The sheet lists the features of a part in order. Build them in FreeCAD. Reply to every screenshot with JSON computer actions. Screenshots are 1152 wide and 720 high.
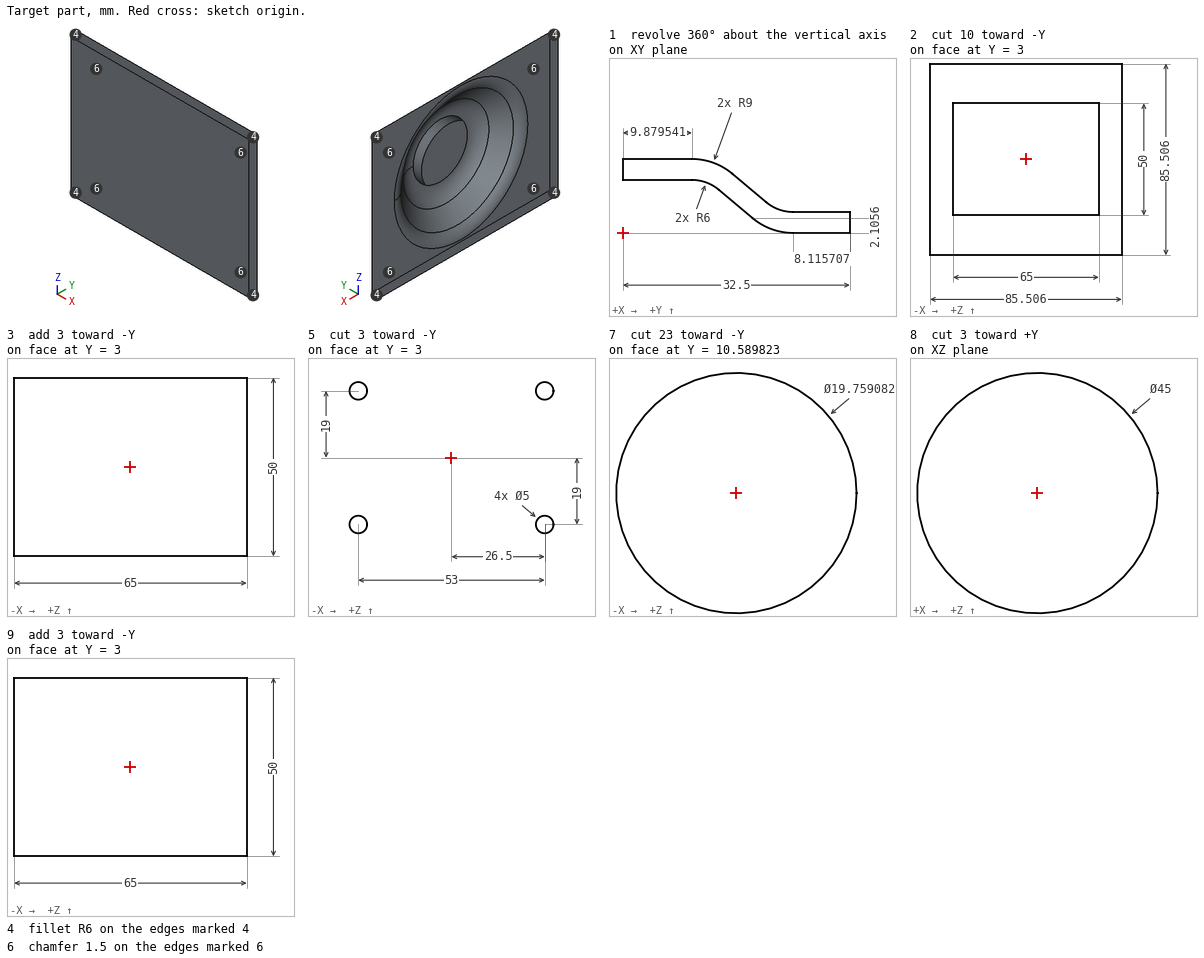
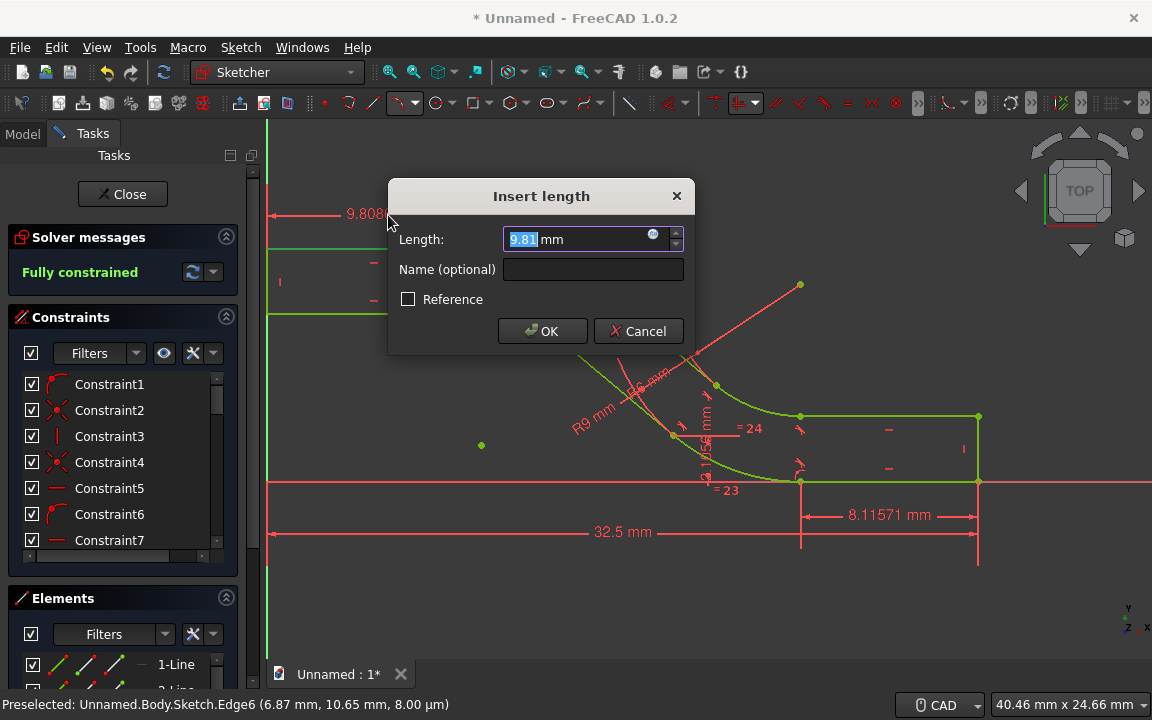
{"action": "type", "text": "9.879541"}
{"action": "key", "text": "Return"}
{"action": "key", "text": "Escape"}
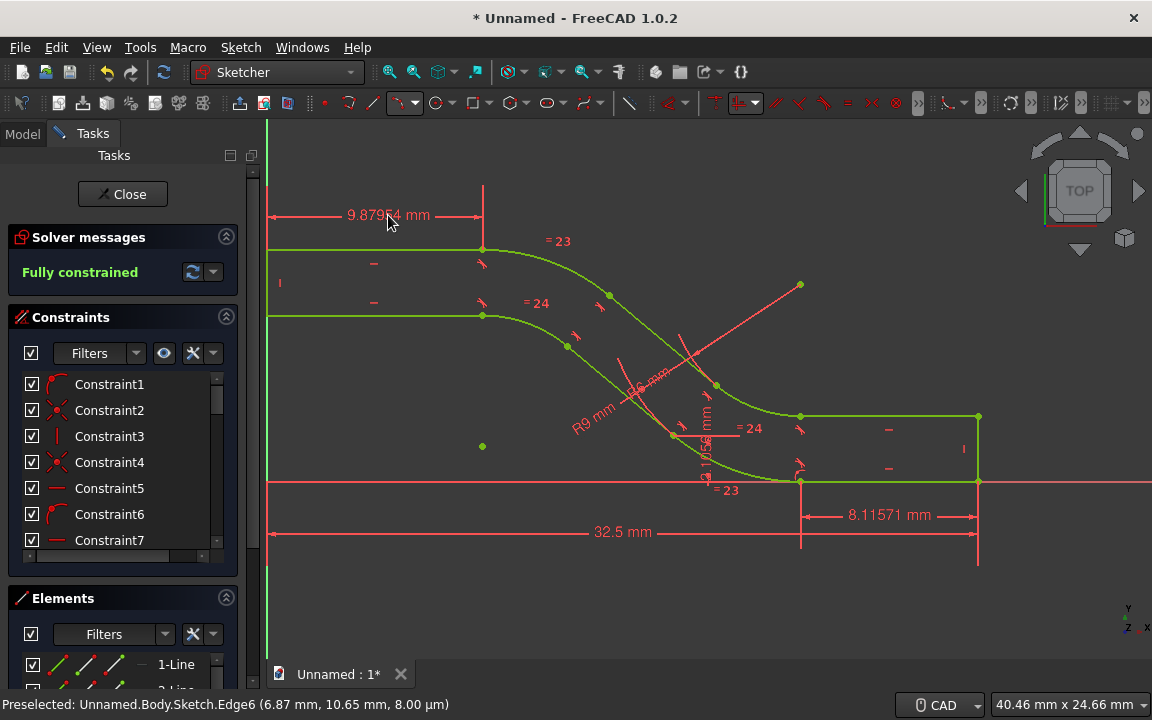
{"action": "left_click", "coordinate": [123, 194]}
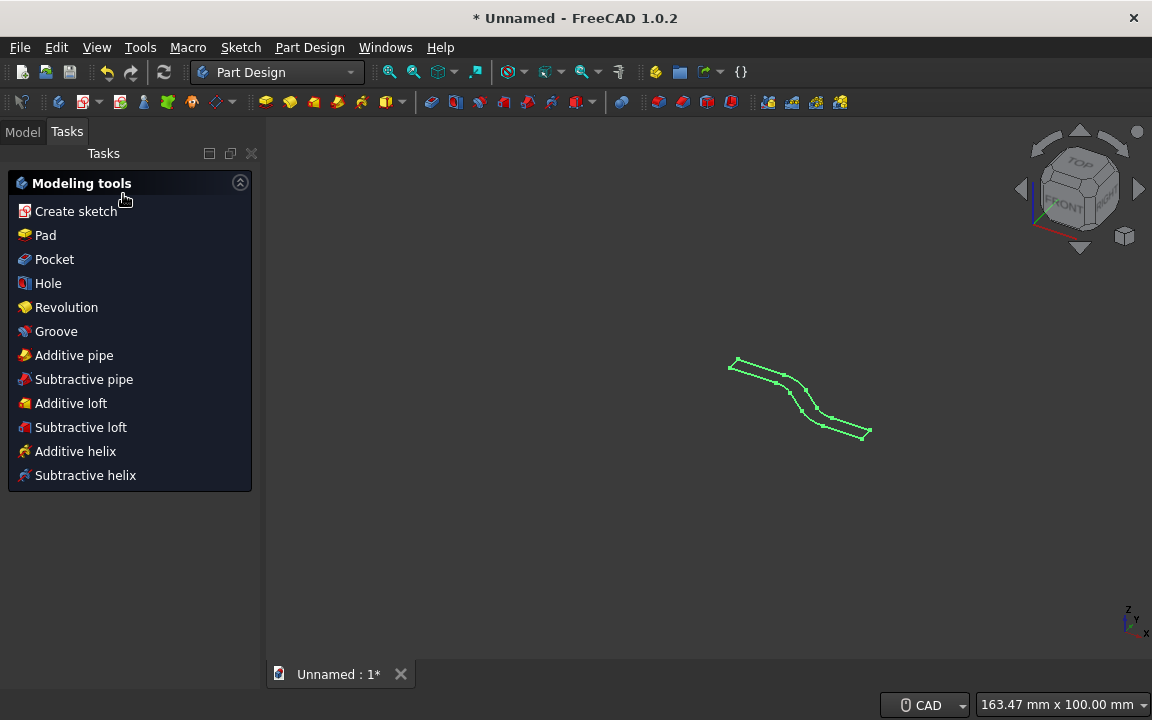
{"action": "left_click", "coordinate": [290, 102]}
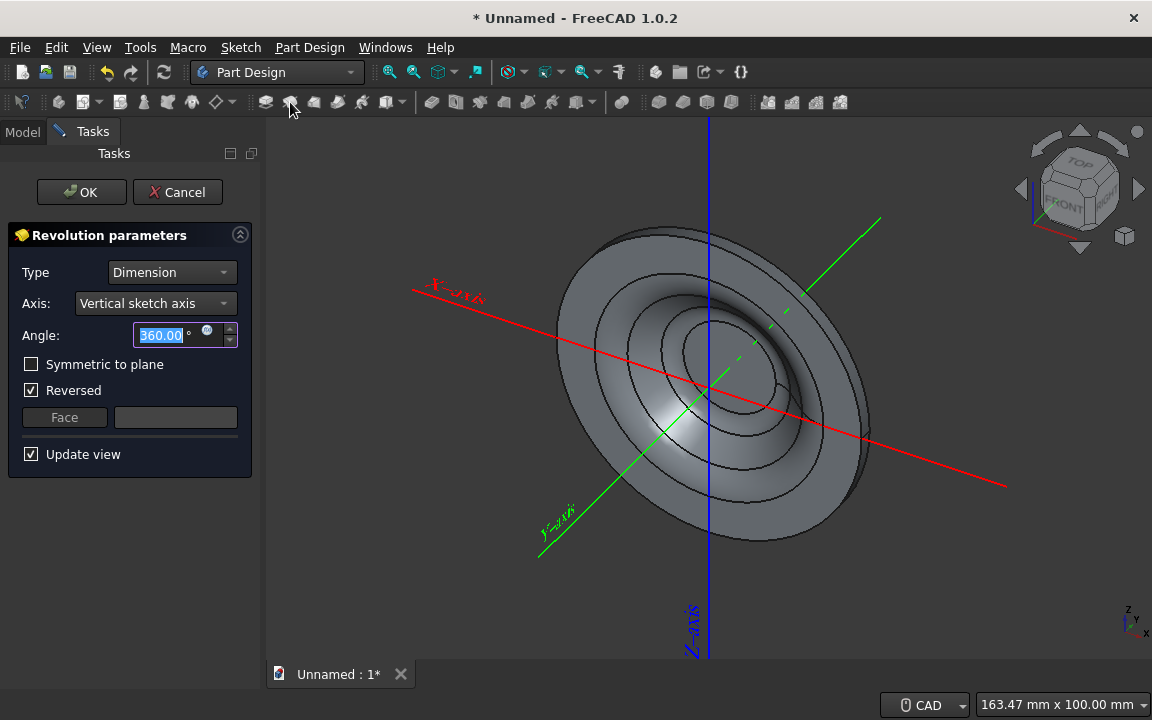
{"action": "left_click", "coordinate": [82, 192]}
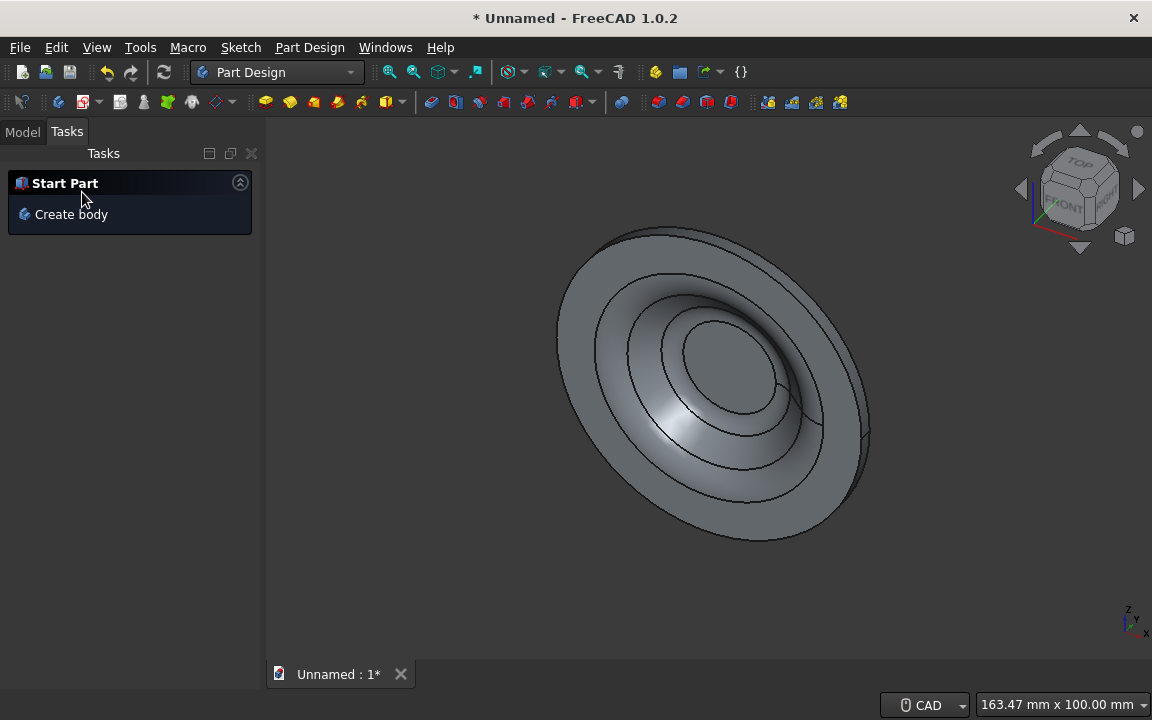
{"action": "key", "text": "4"}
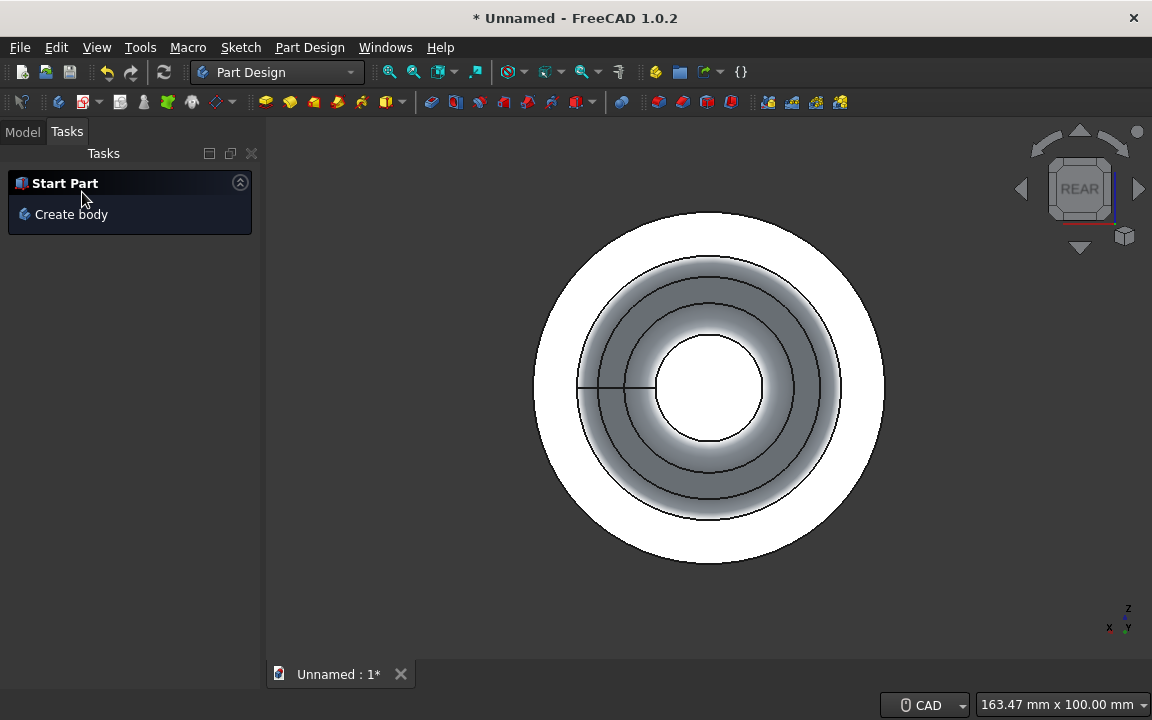
{"action": "left_click", "coordinate": [709, 538]}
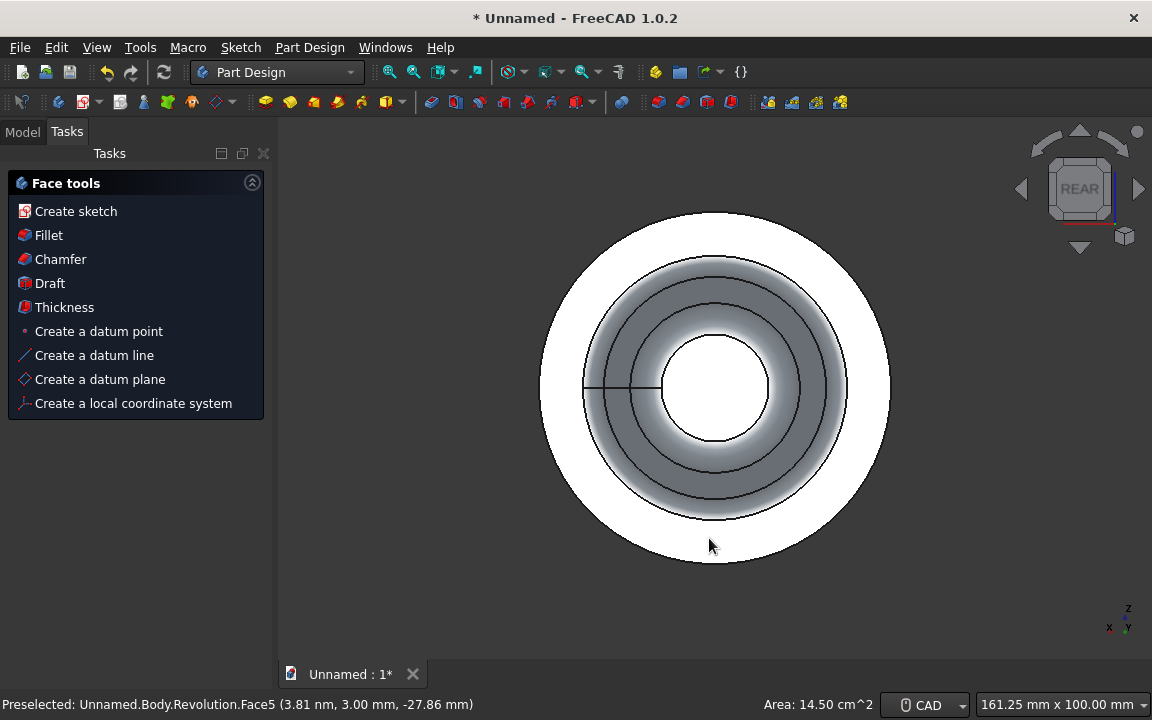
{"action": "left_click", "coordinate": [84, 102]}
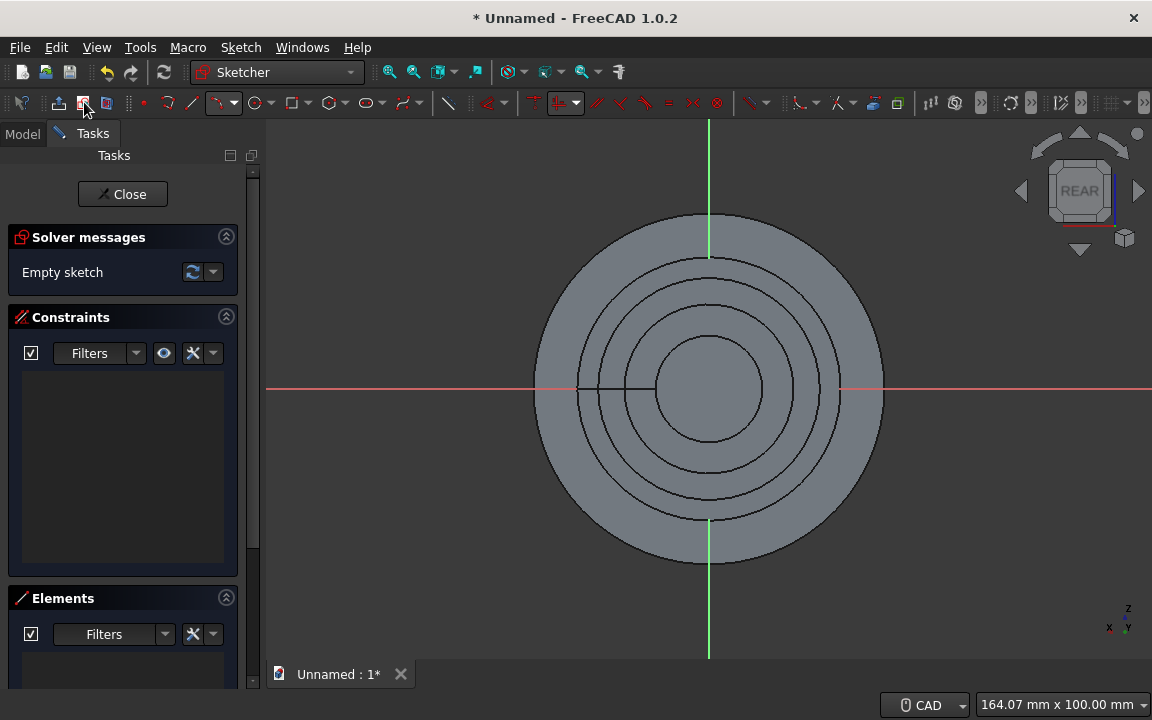
{"action": "left_click", "coordinate": [108, 104]}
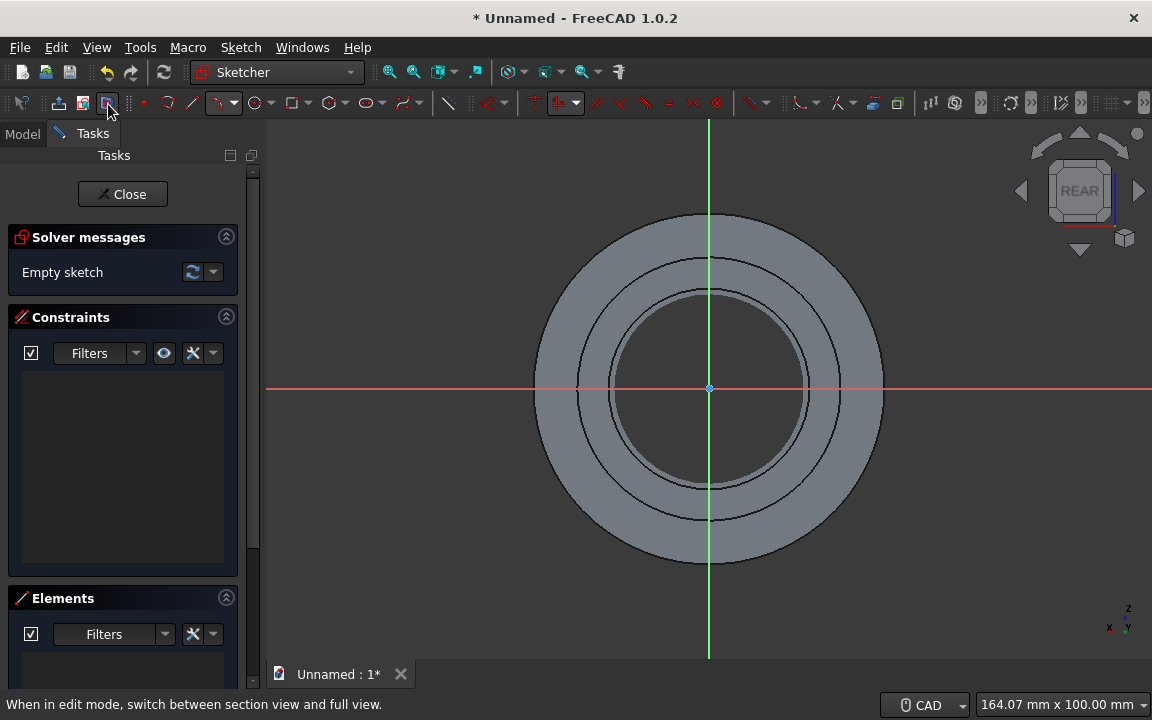
{"action": "scroll", "coordinate": [501, 389], "scroll_direction": "down", "scroll_amount": 2}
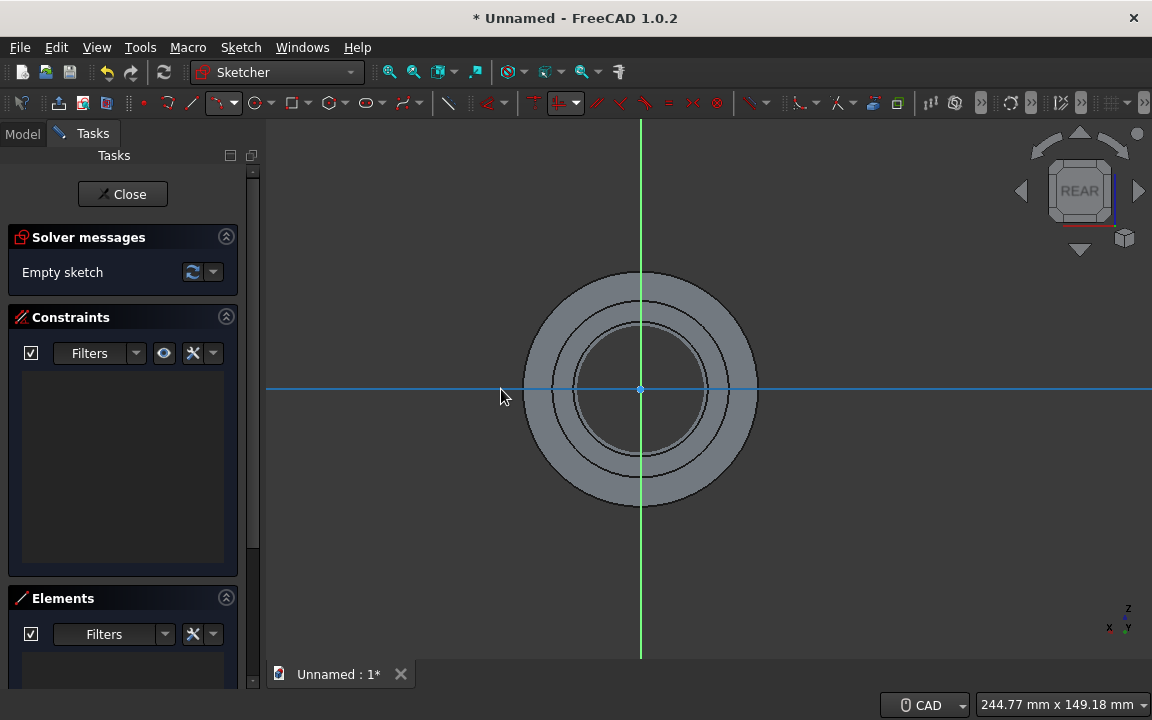
{"action": "left_click", "coordinate": [310, 104]}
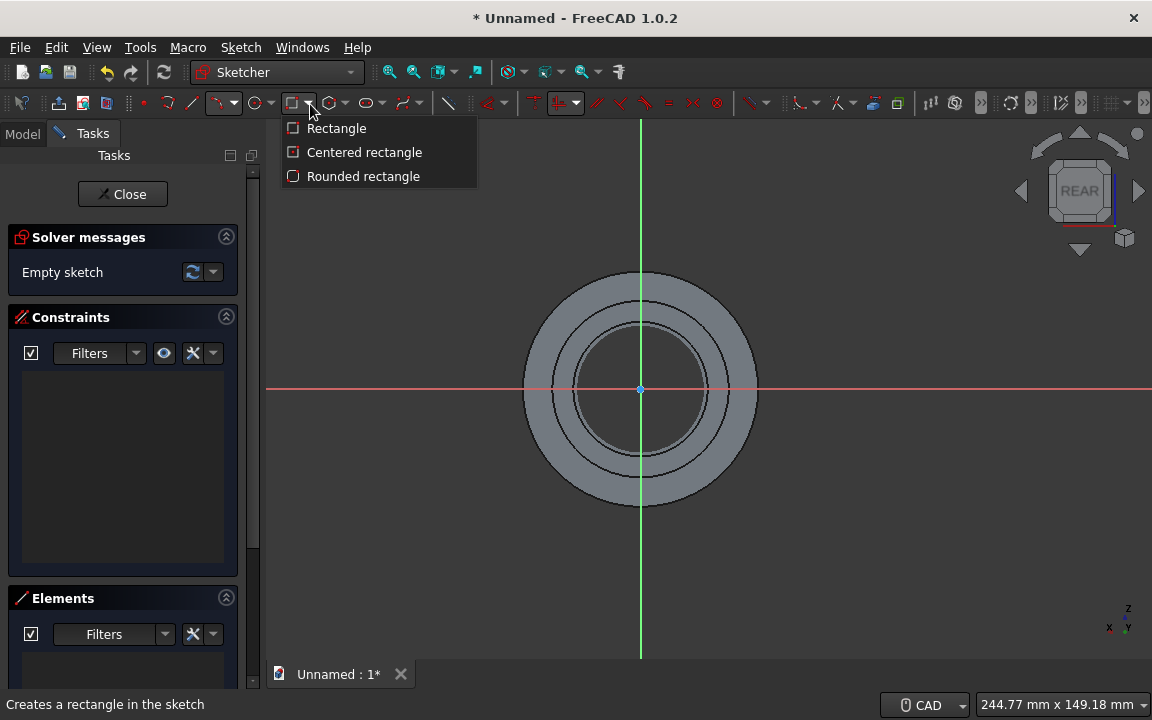
{"action": "left_click", "coordinate": [380, 152]}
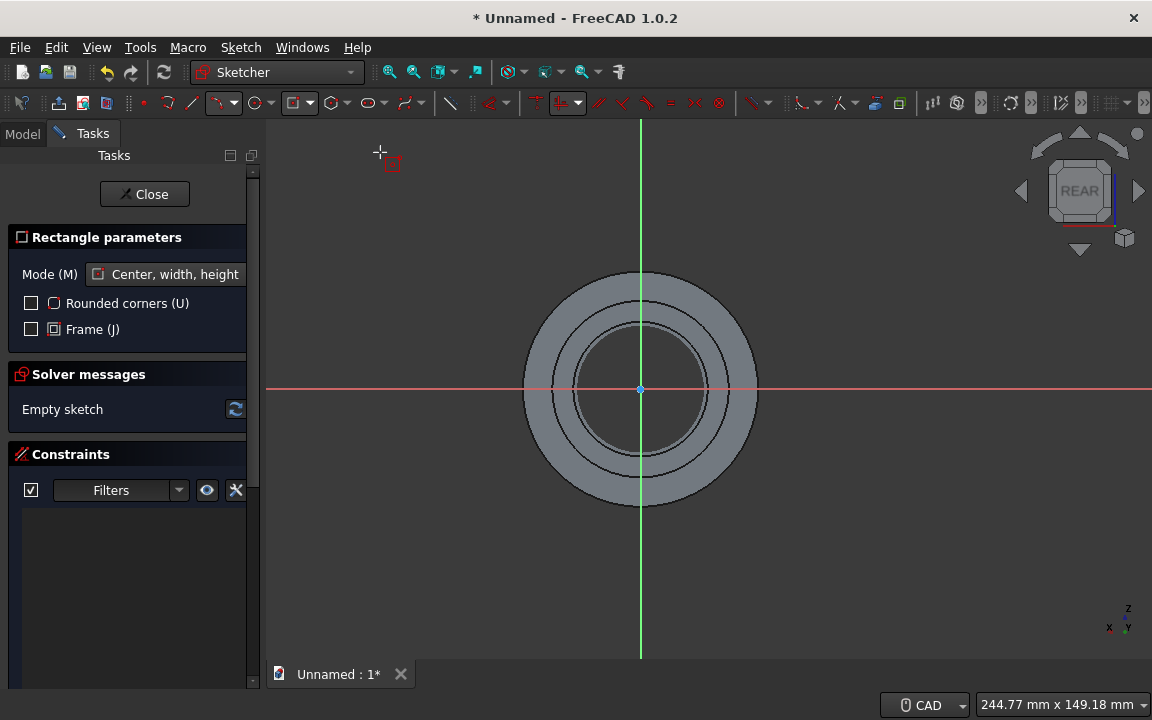
{"action": "left_click", "coordinate": [641, 389]}
{"action": "left_click", "coordinate": [795, 234]}